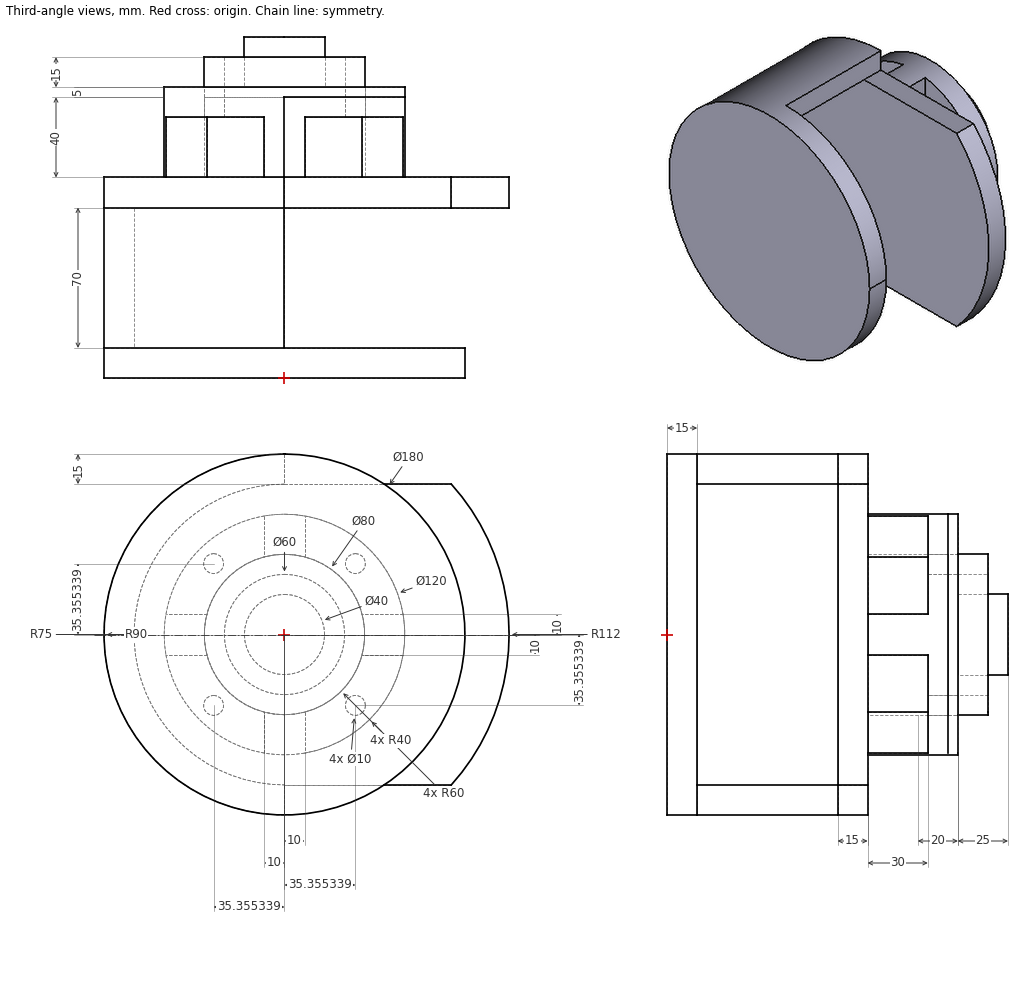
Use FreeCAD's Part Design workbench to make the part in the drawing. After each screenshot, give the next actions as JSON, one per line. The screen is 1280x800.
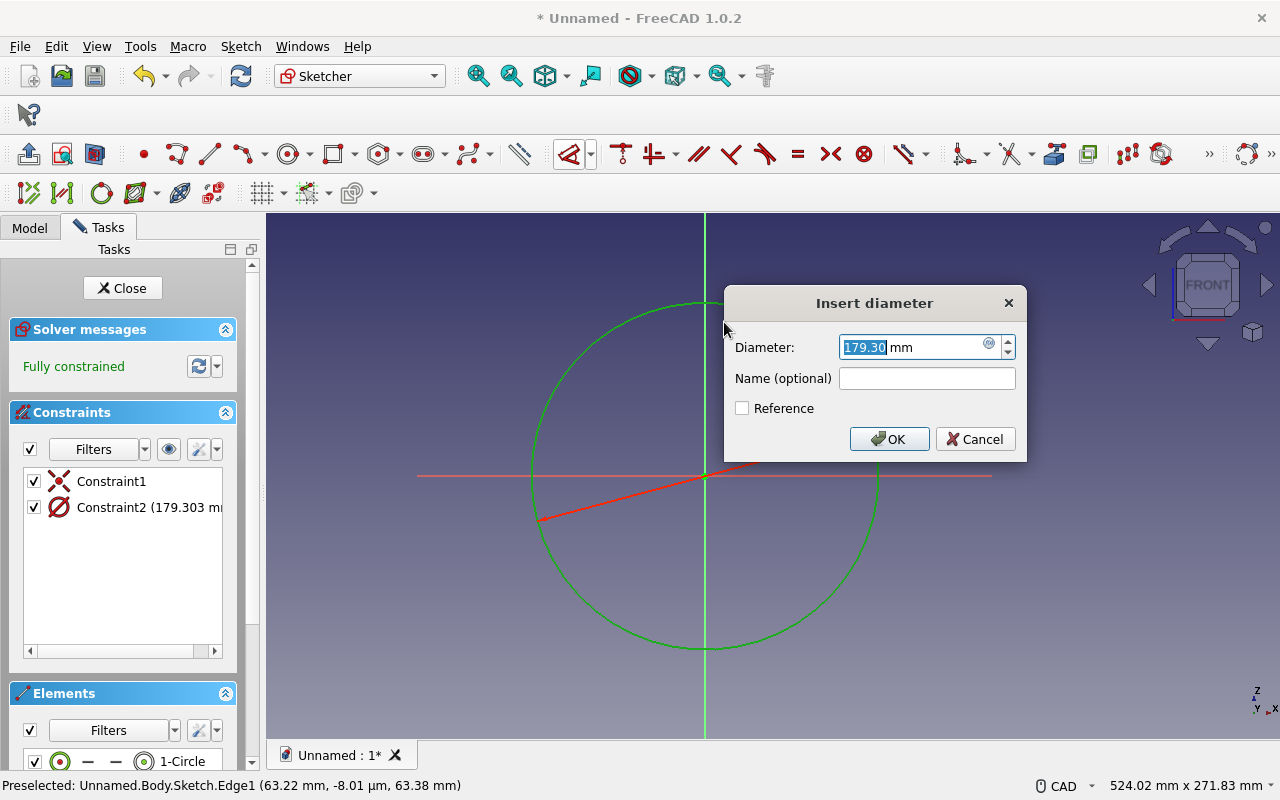
{"action": "type", "text": "180"}
{"action": "key", "text": "Return"}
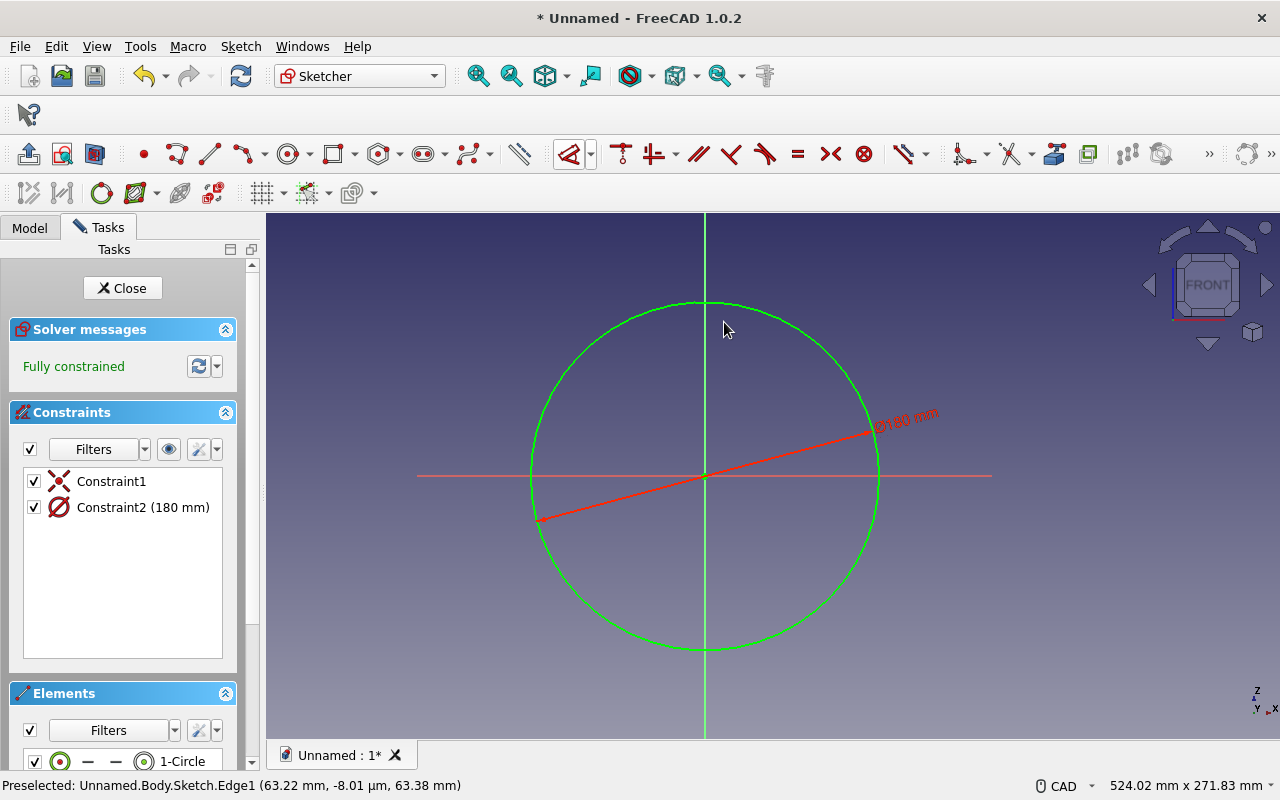
{"action": "left_click", "coordinate": [123, 288]}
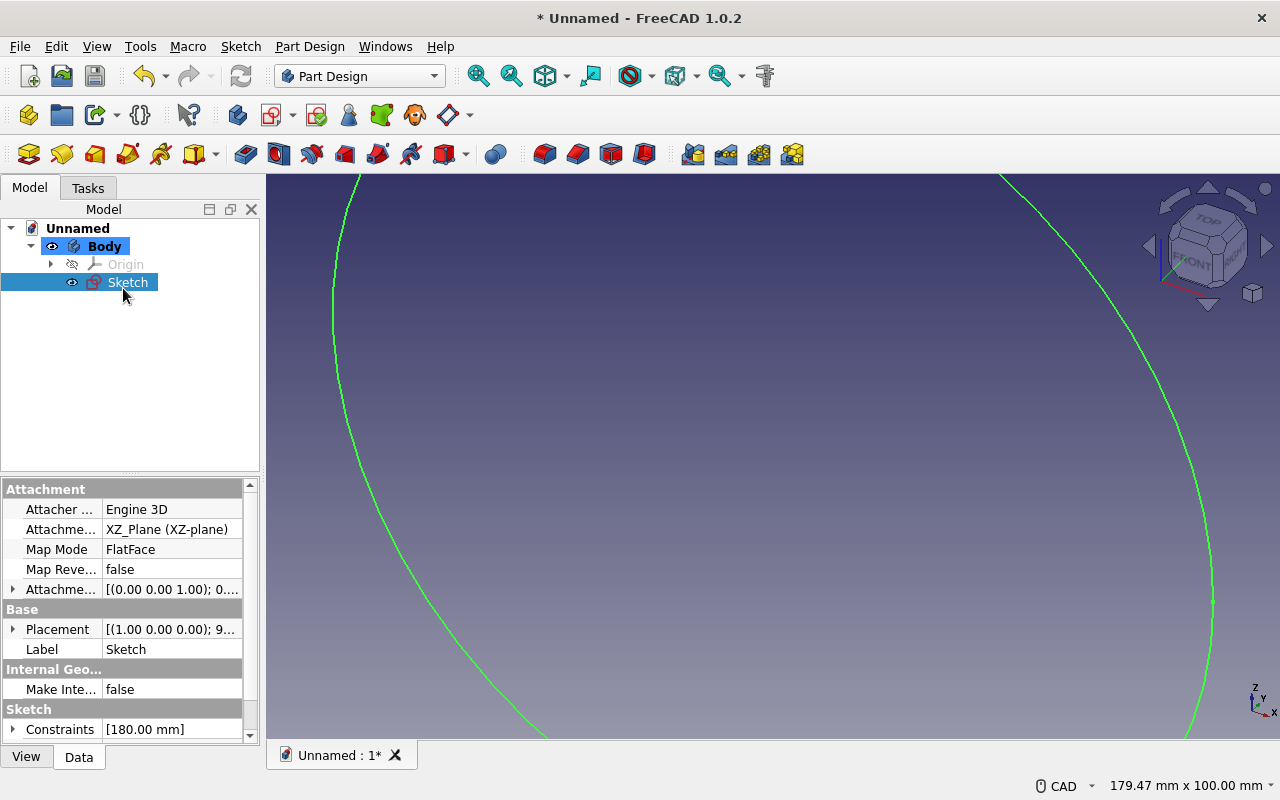
{"action": "left_click", "coordinate": [29, 154]}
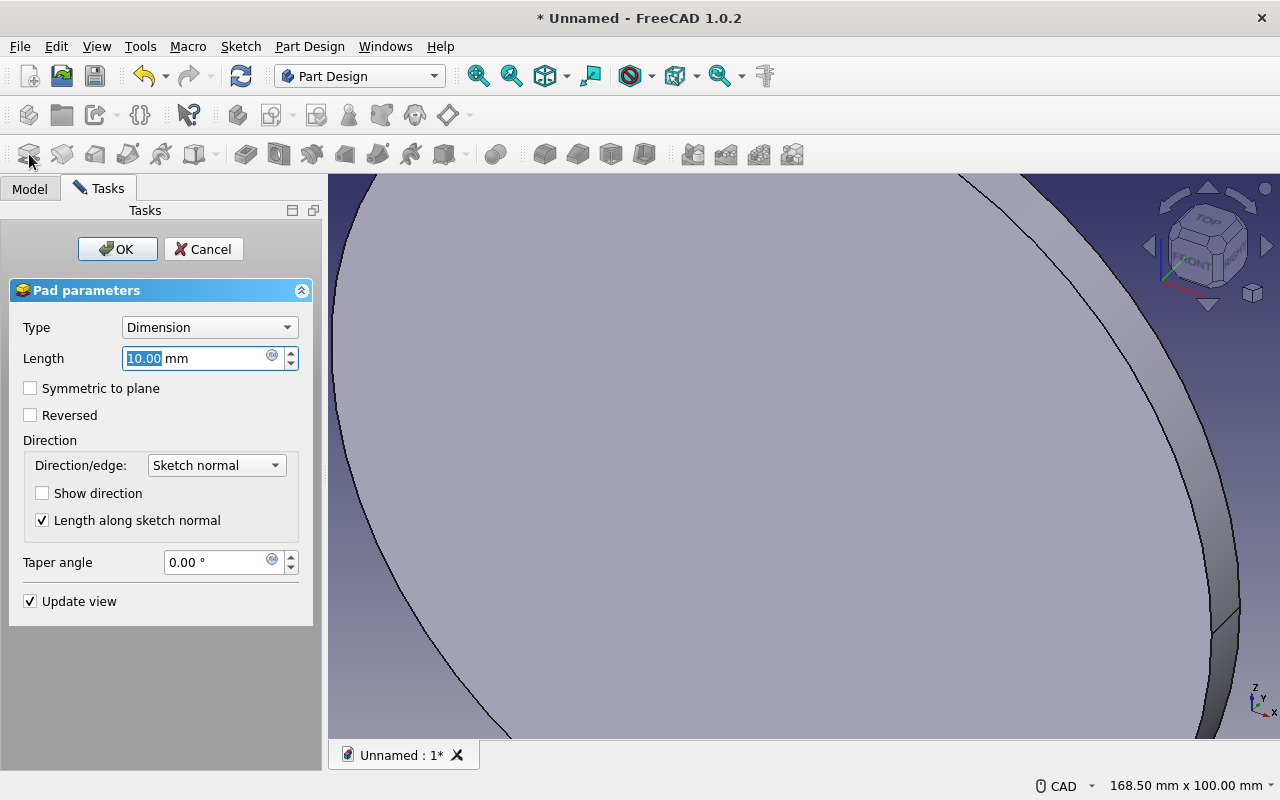
{"action": "type", "text": "15"}
{"action": "key", "text": "Tab"}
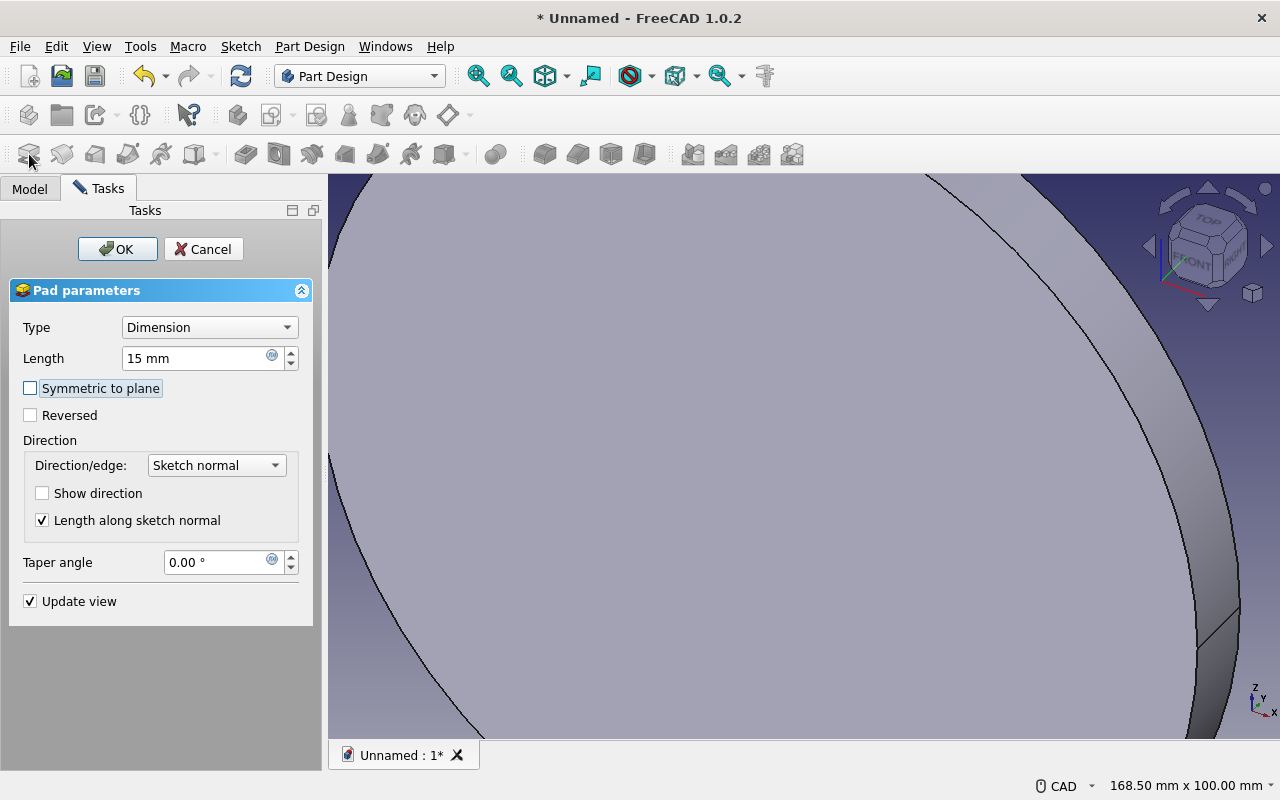
{"action": "left_click", "coordinate": [31, 415]}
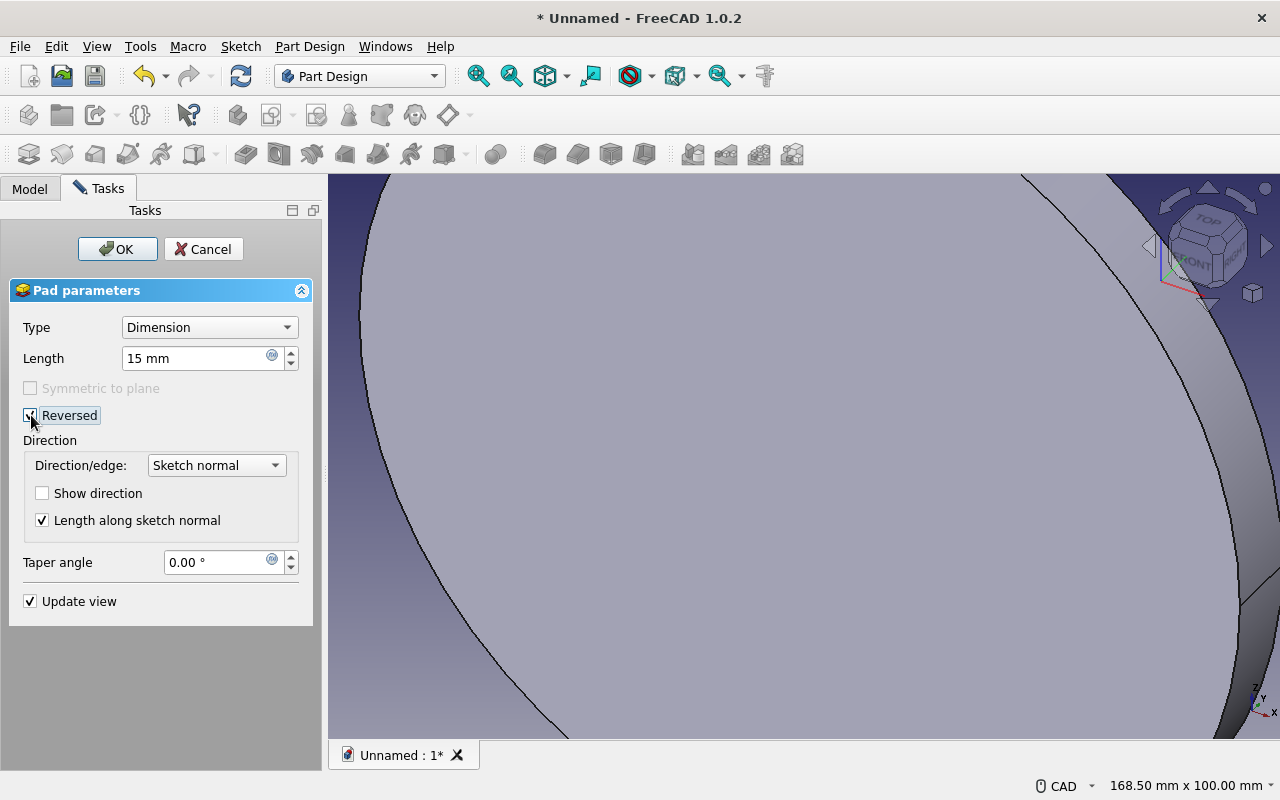
{"action": "left_click", "coordinate": [118, 249]}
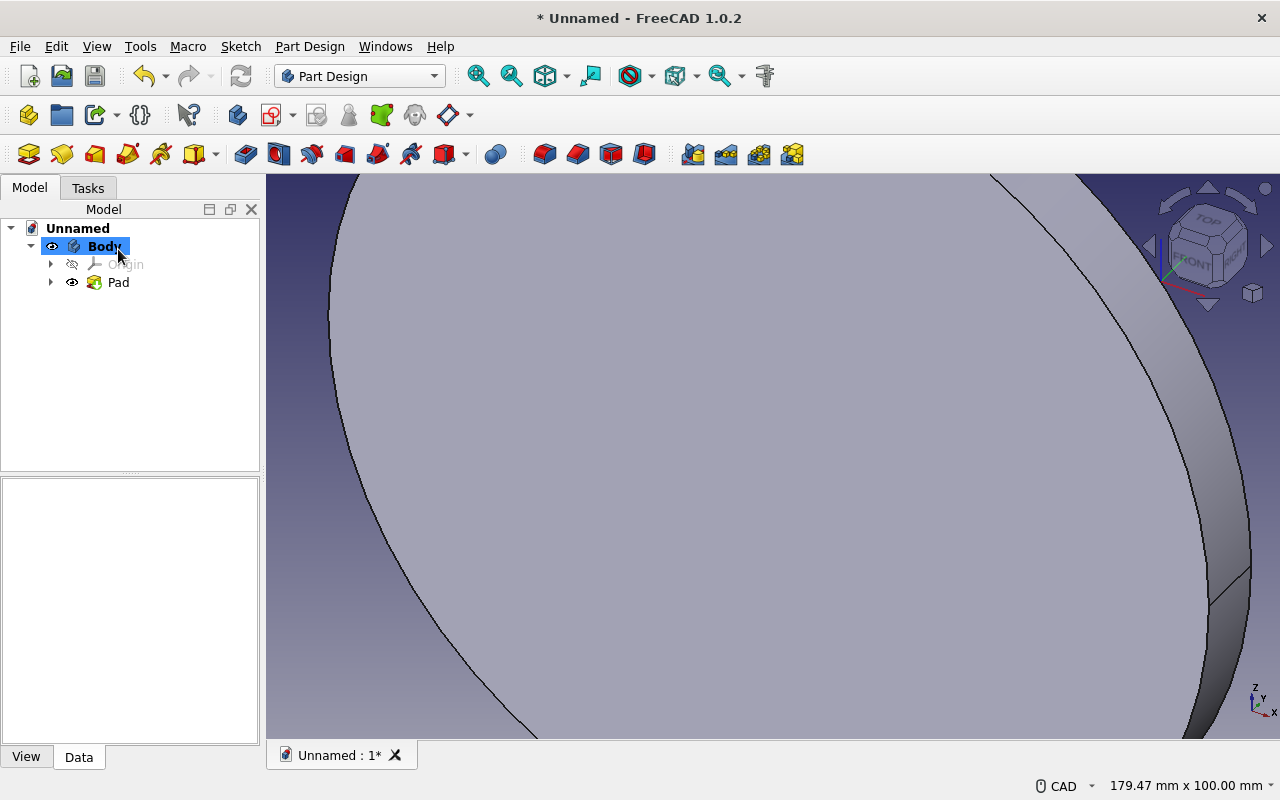
{"action": "left_click", "coordinate": [479, 76]}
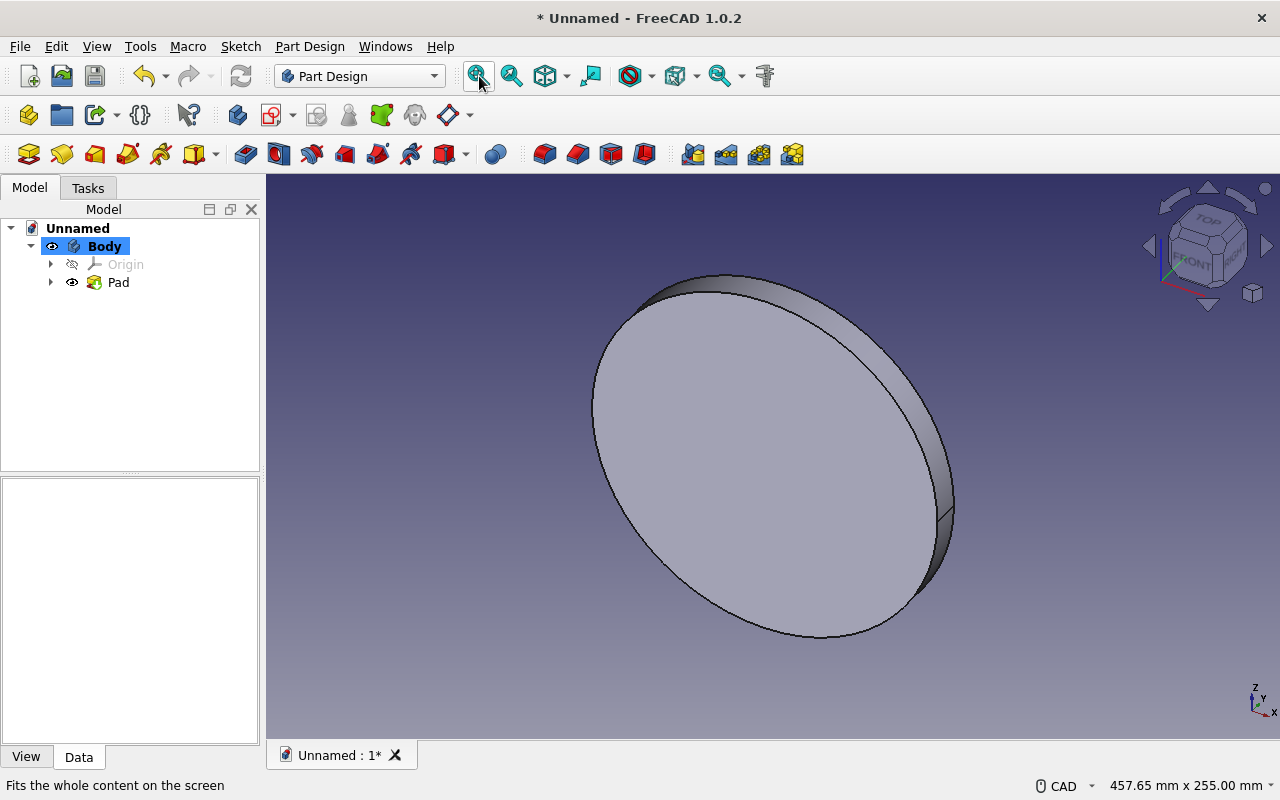
{"action": "key", "text": "4"}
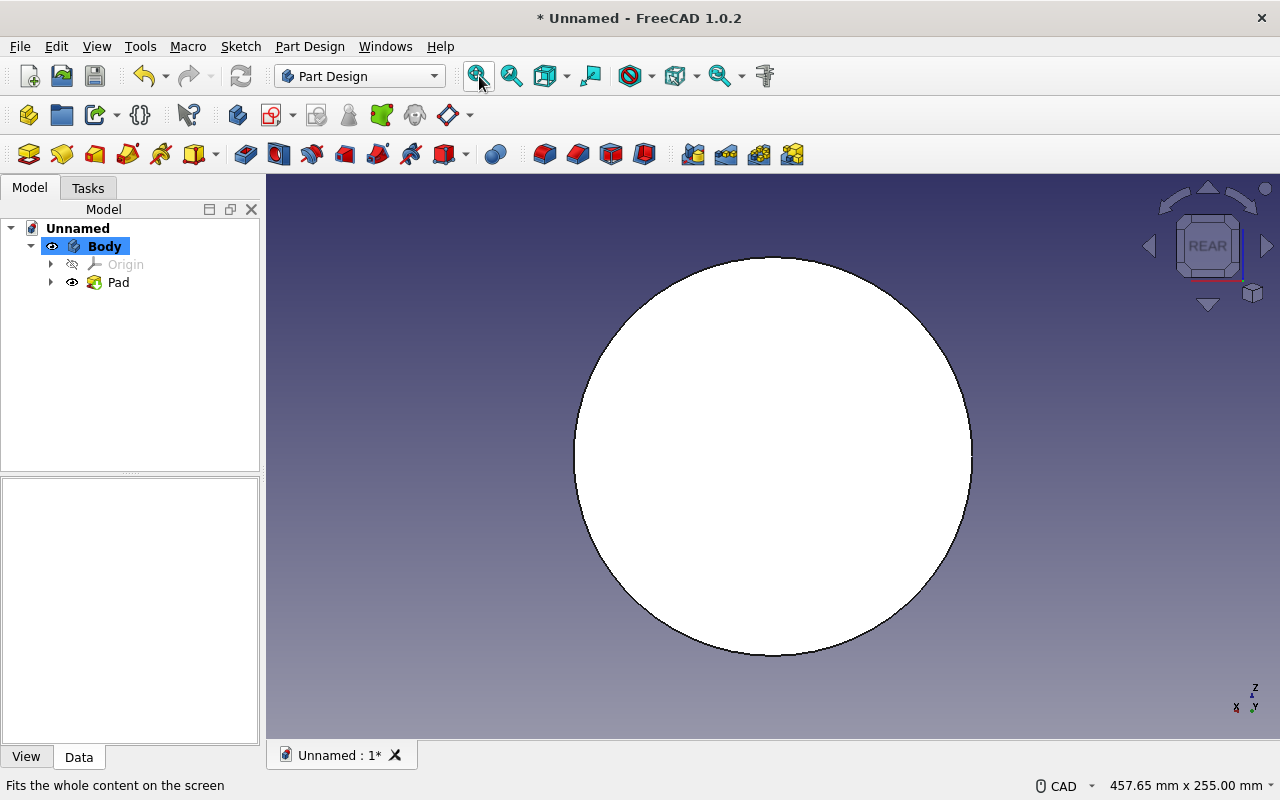
{"action": "left_click", "coordinate": [773, 455]}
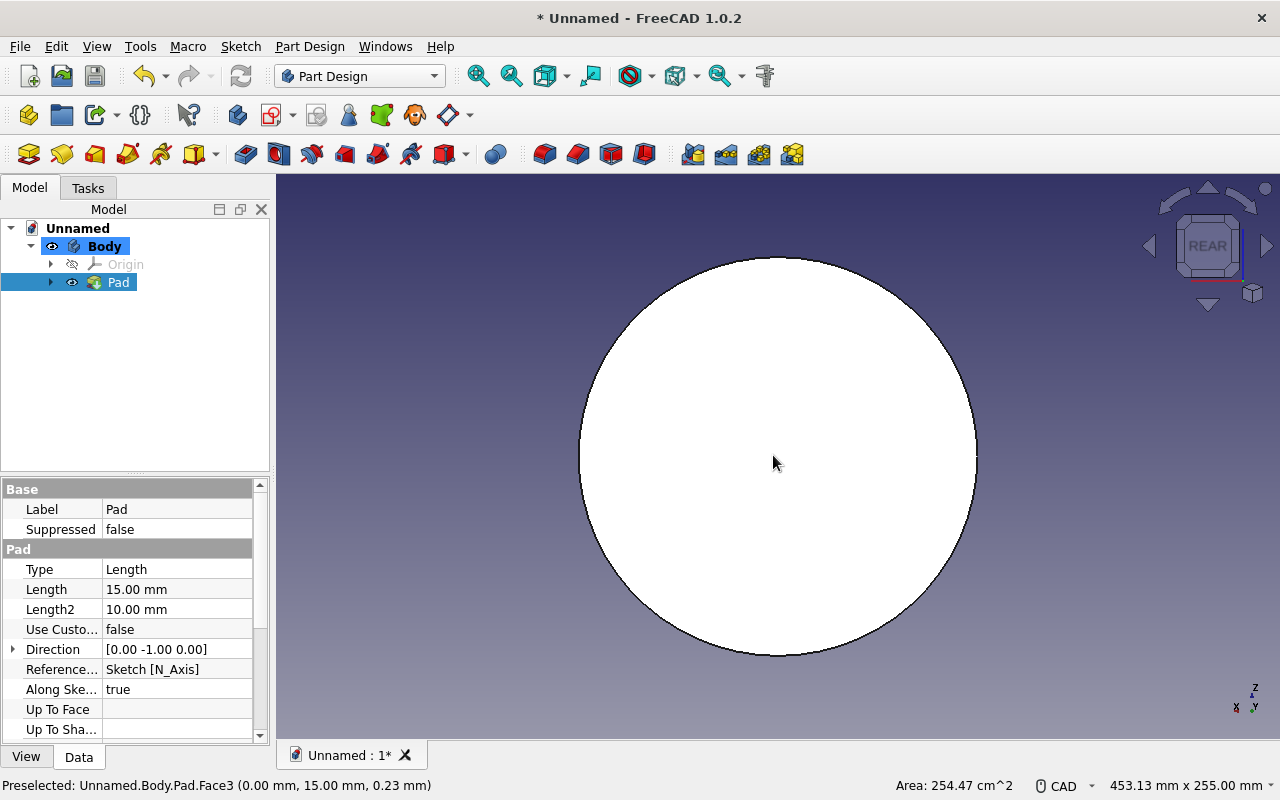
{"action": "left_click", "coordinate": [270, 116]}